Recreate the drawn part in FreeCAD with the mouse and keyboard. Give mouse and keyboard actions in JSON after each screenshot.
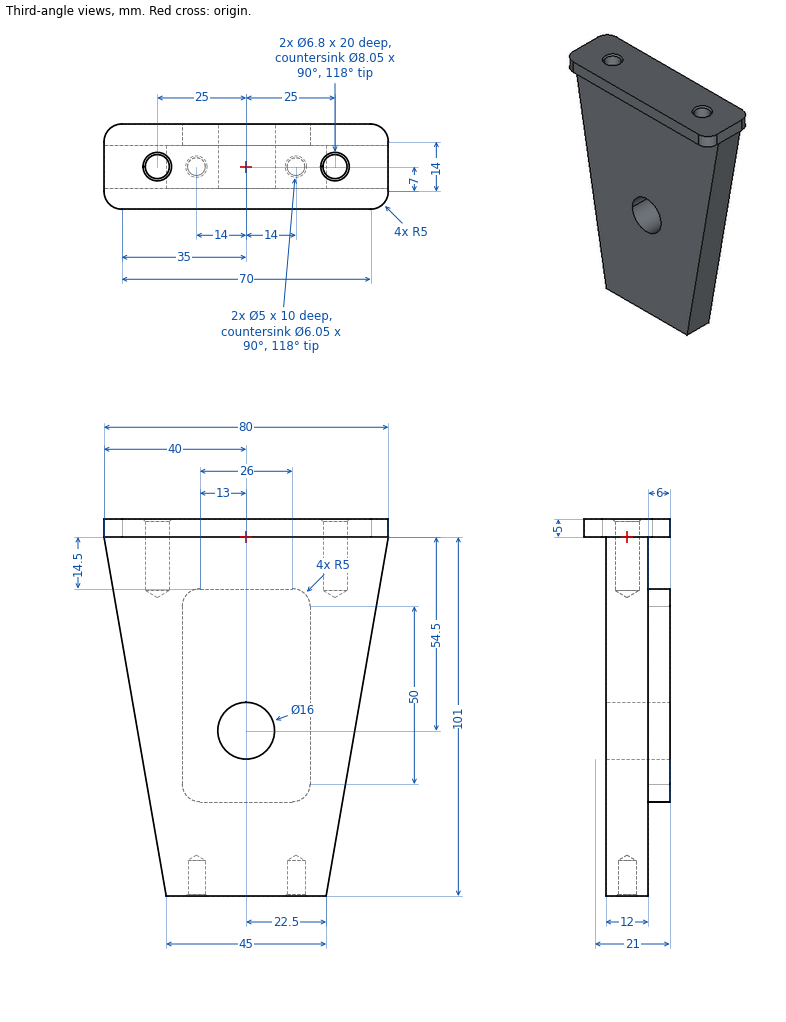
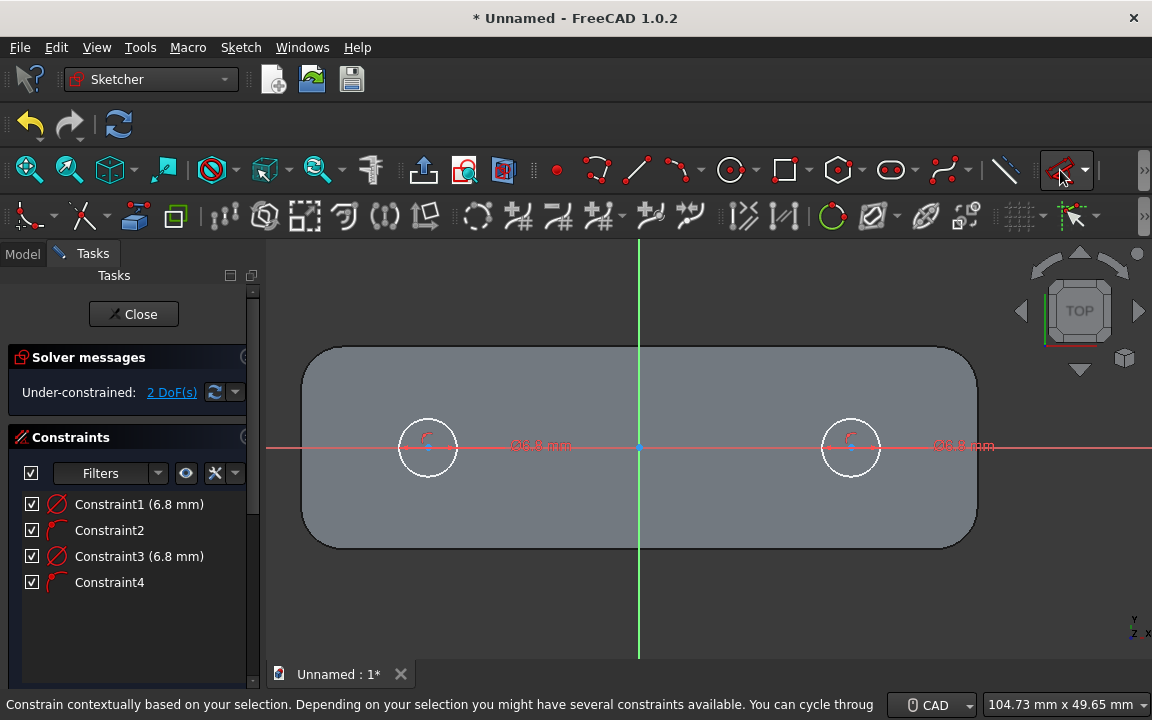
{"action": "left_click", "coordinate": [851, 448]}
{"action": "left_click", "coordinate": [745, 482]}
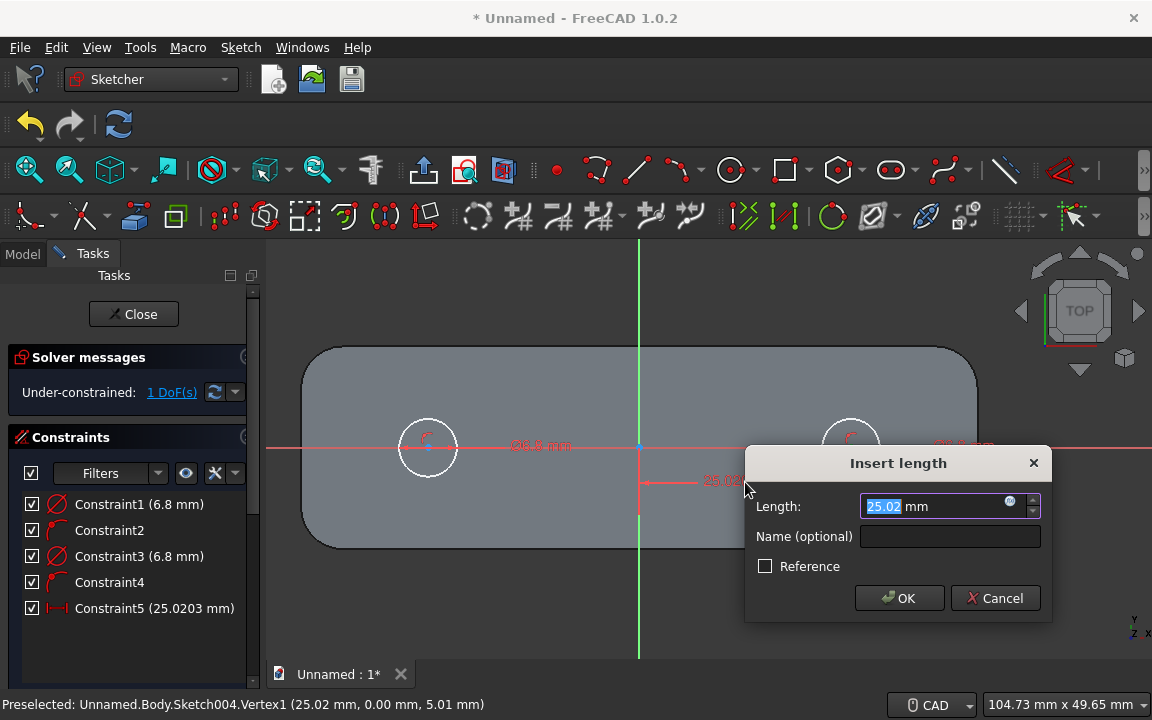
{"action": "type", "text": "25"}
{"action": "key", "text": "Return"}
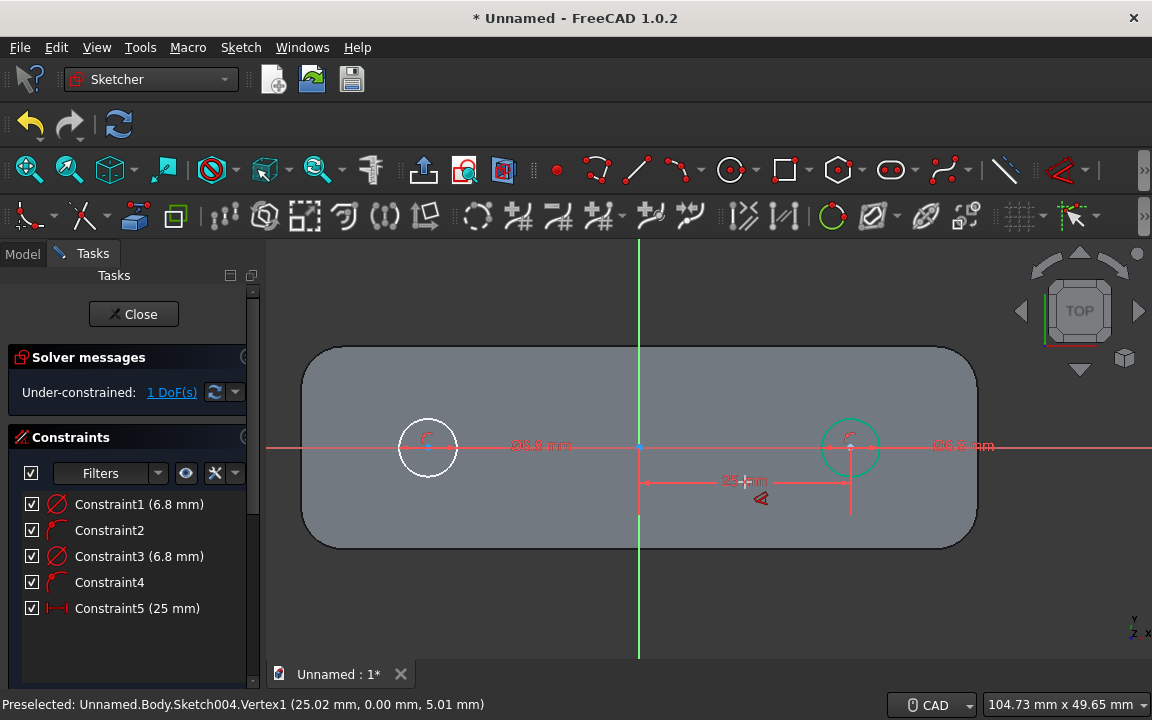
{"action": "left_click", "coordinate": [428, 448]}
{"action": "left_click", "coordinate": [534, 482]}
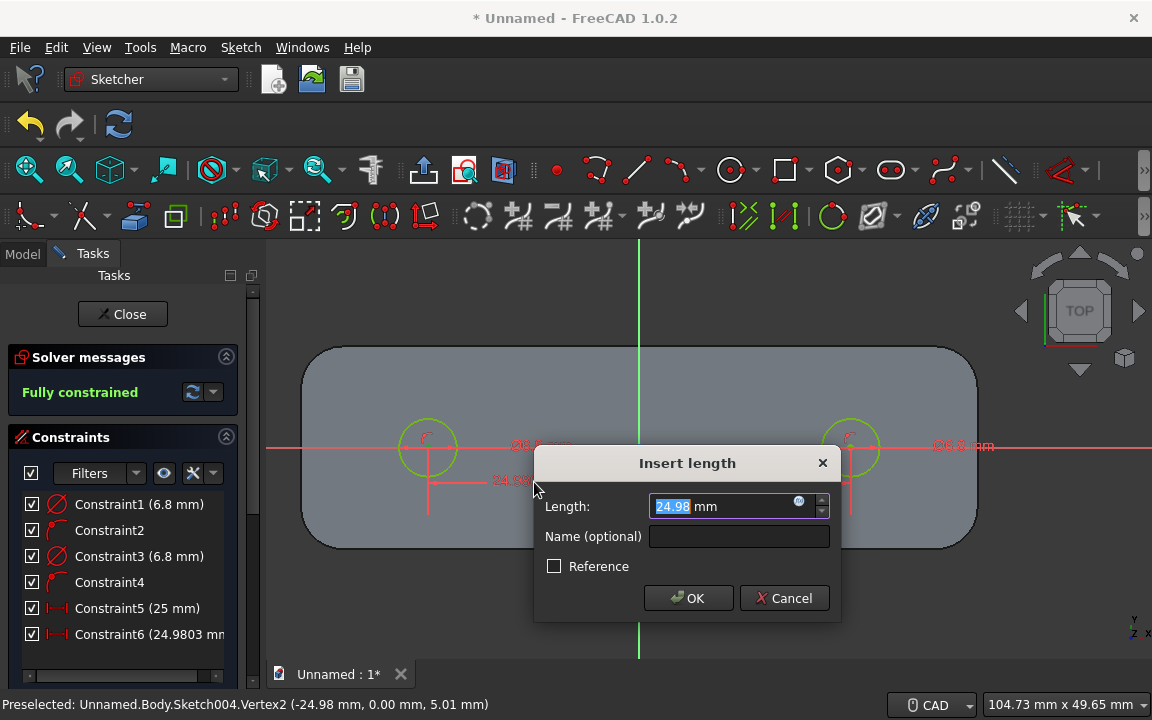
{"action": "type", "text": "25"}
{"action": "key", "text": "Return"}
{"action": "key", "text": "Escape"}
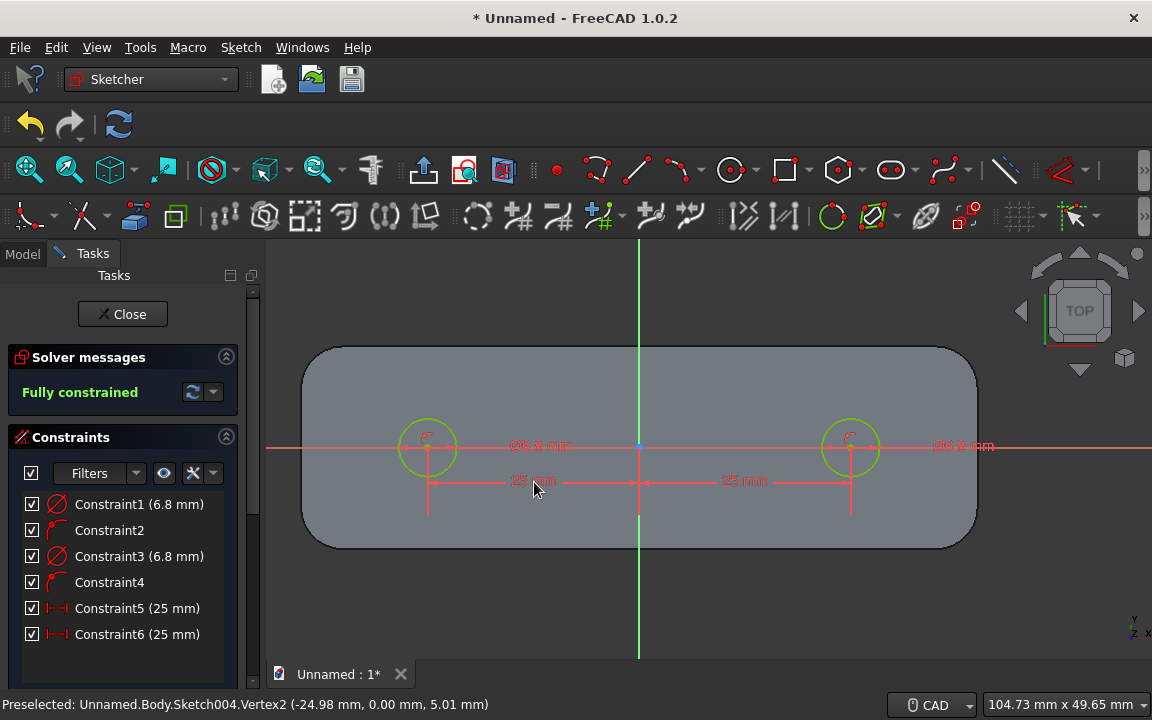
{"action": "left_click", "coordinate": [123, 314]}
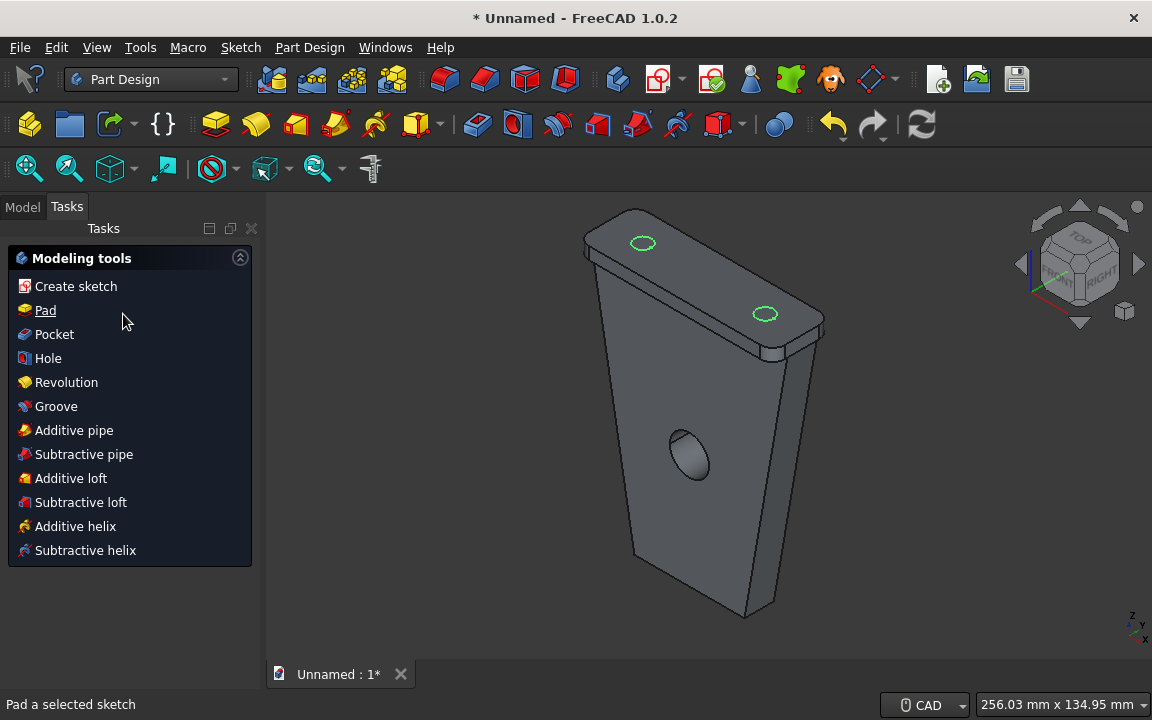
{"action": "left_click", "coordinate": [518, 124]}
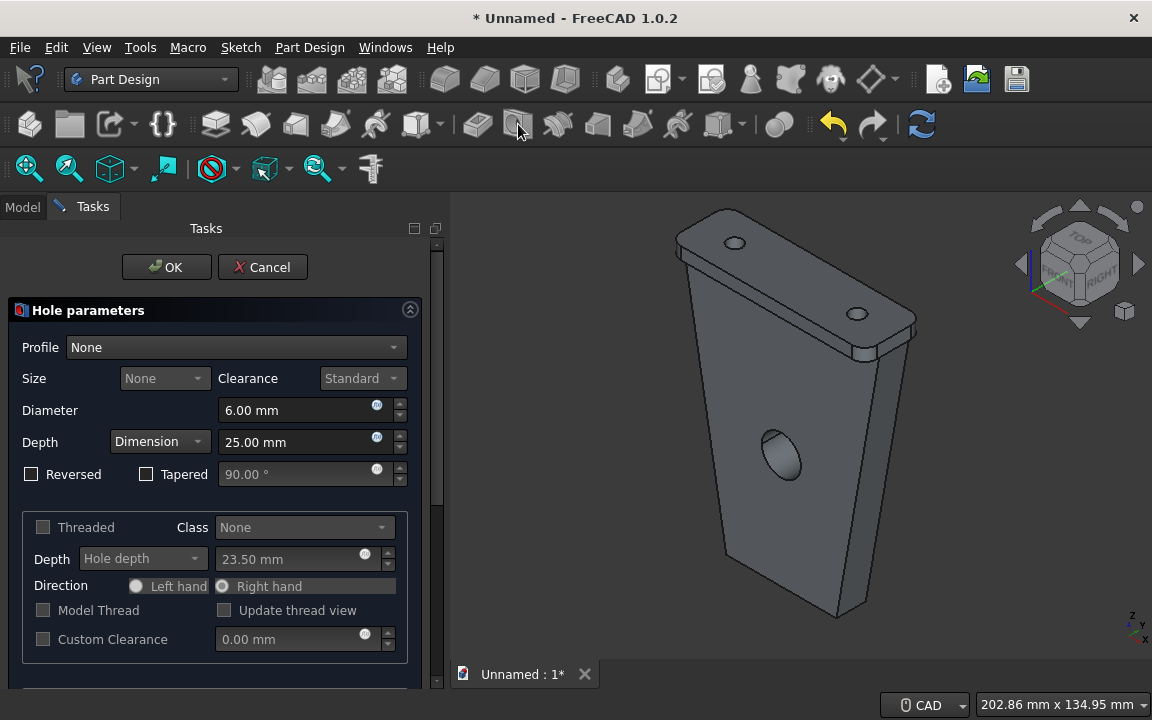
{"action": "triple_click", "coordinate": [305, 410]}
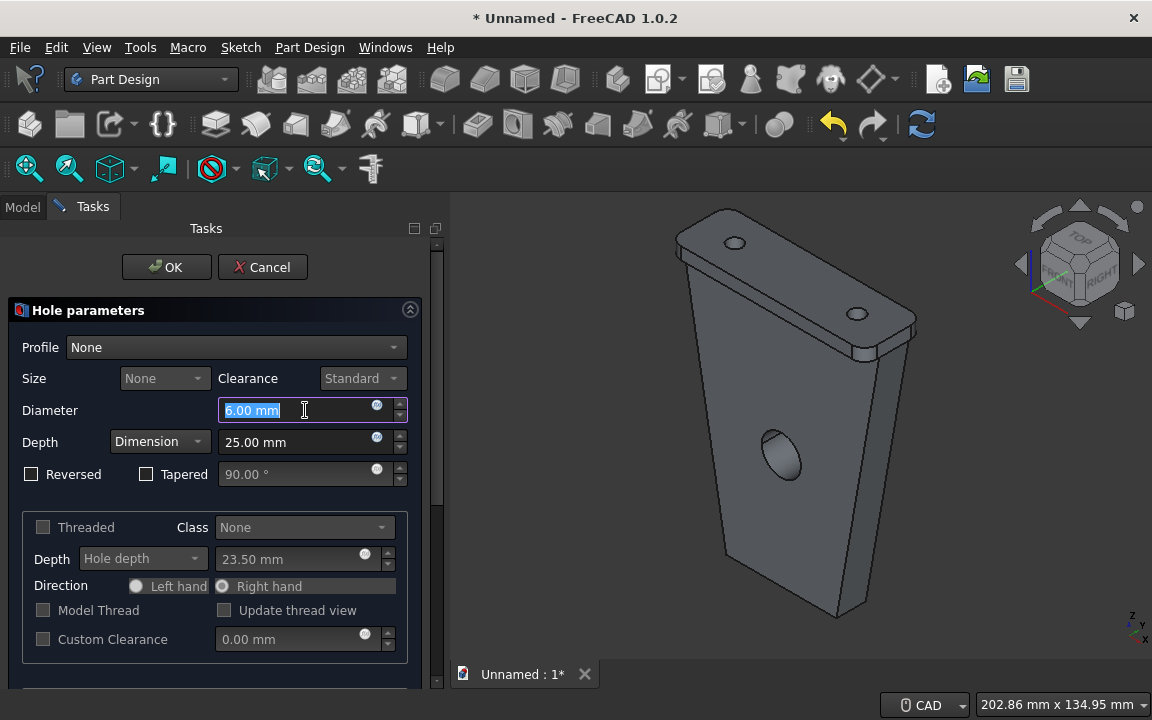
{"action": "type", "text": "6.8"}
{"action": "key", "text": "Tab"}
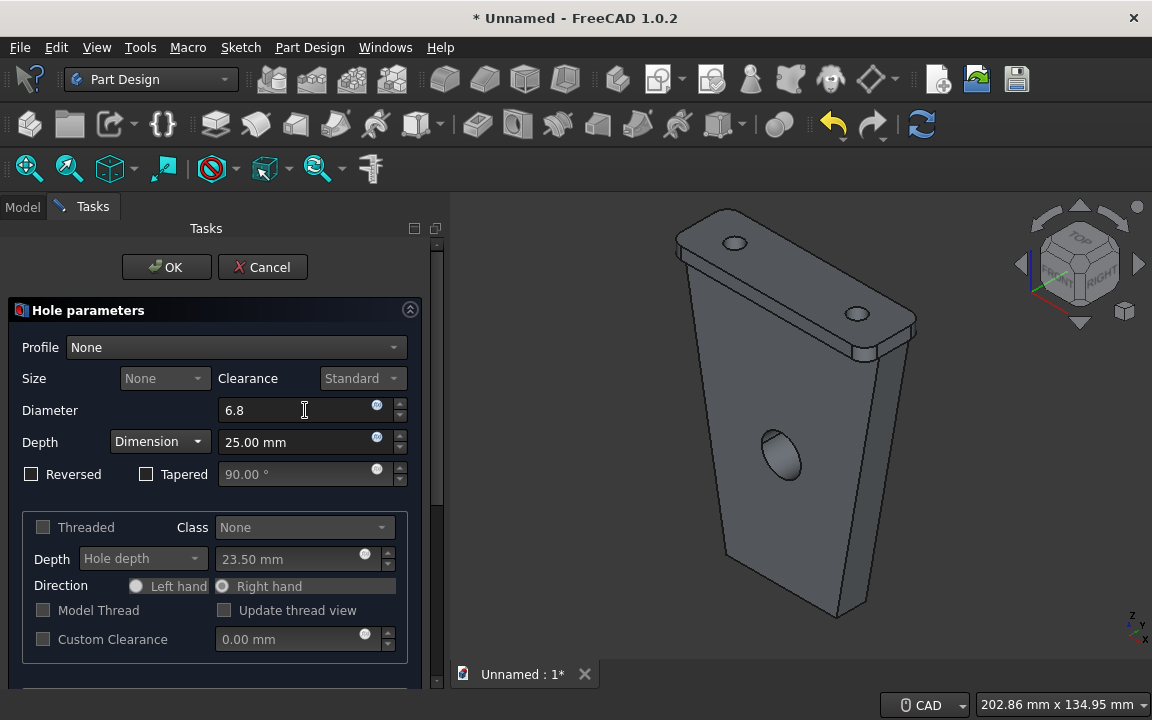
{"action": "triple_click", "coordinate": [305, 442]}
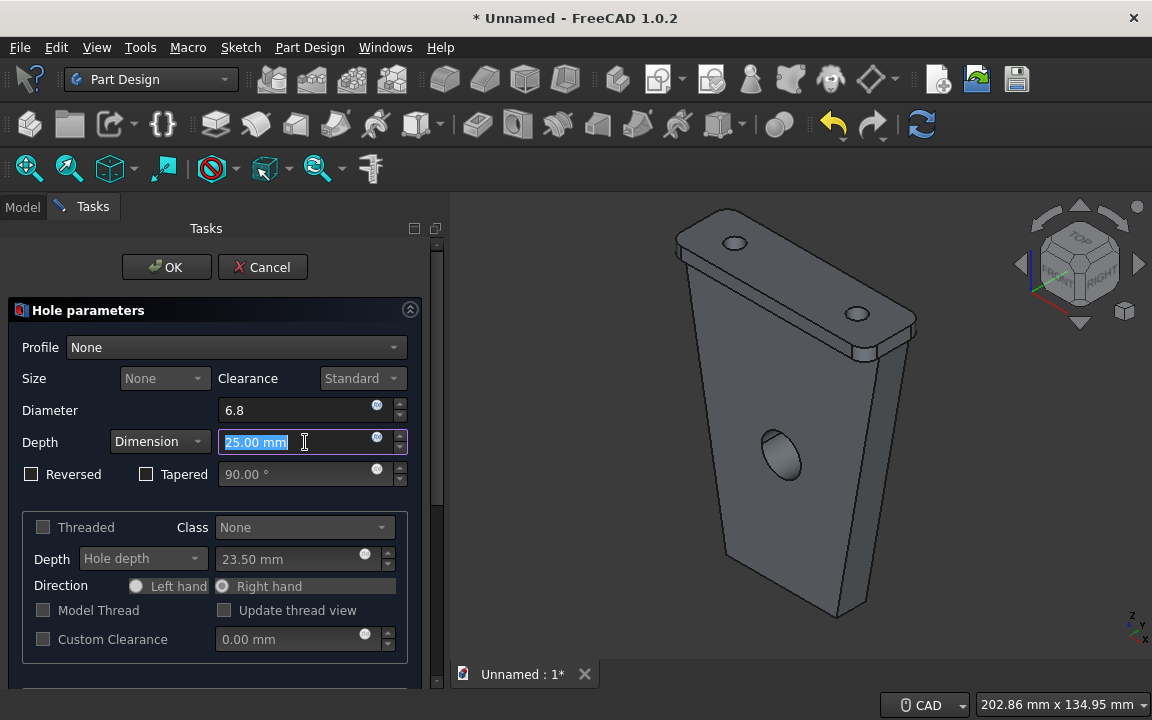
{"action": "type", "text": "20"}
{"action": "key", "text": "Tab"}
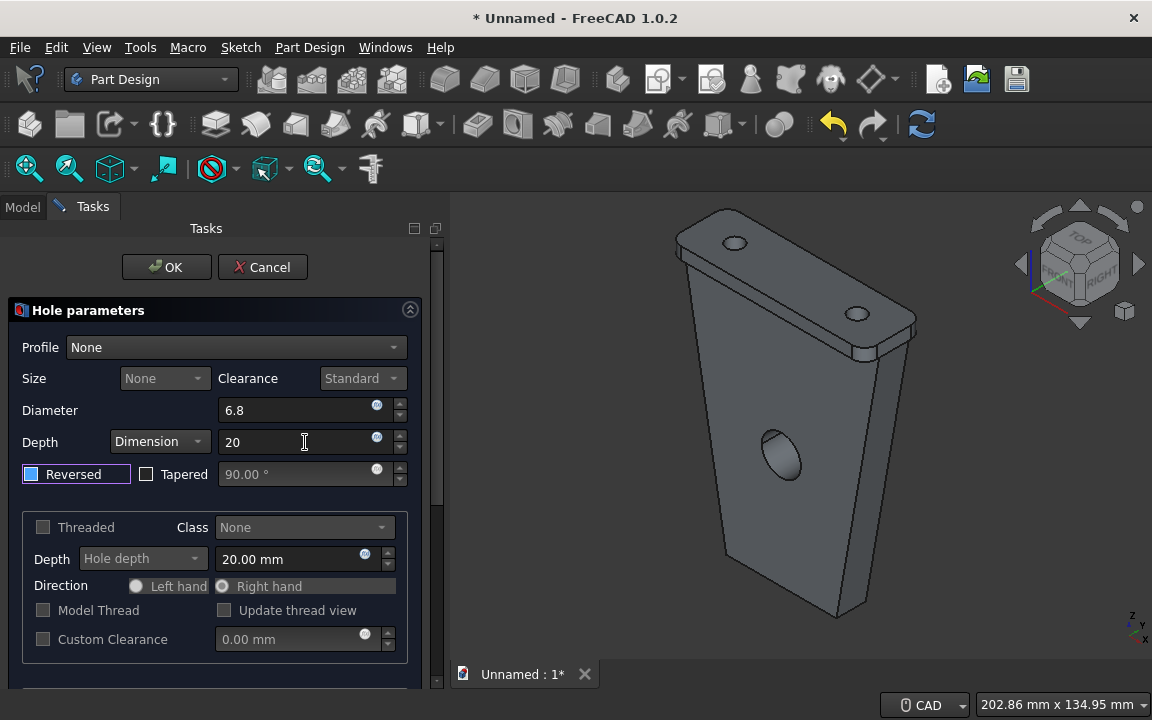
{"action": "scroll", "coordinate": [437, 463], "scroll_direction": "down", "scroll_amount": 2}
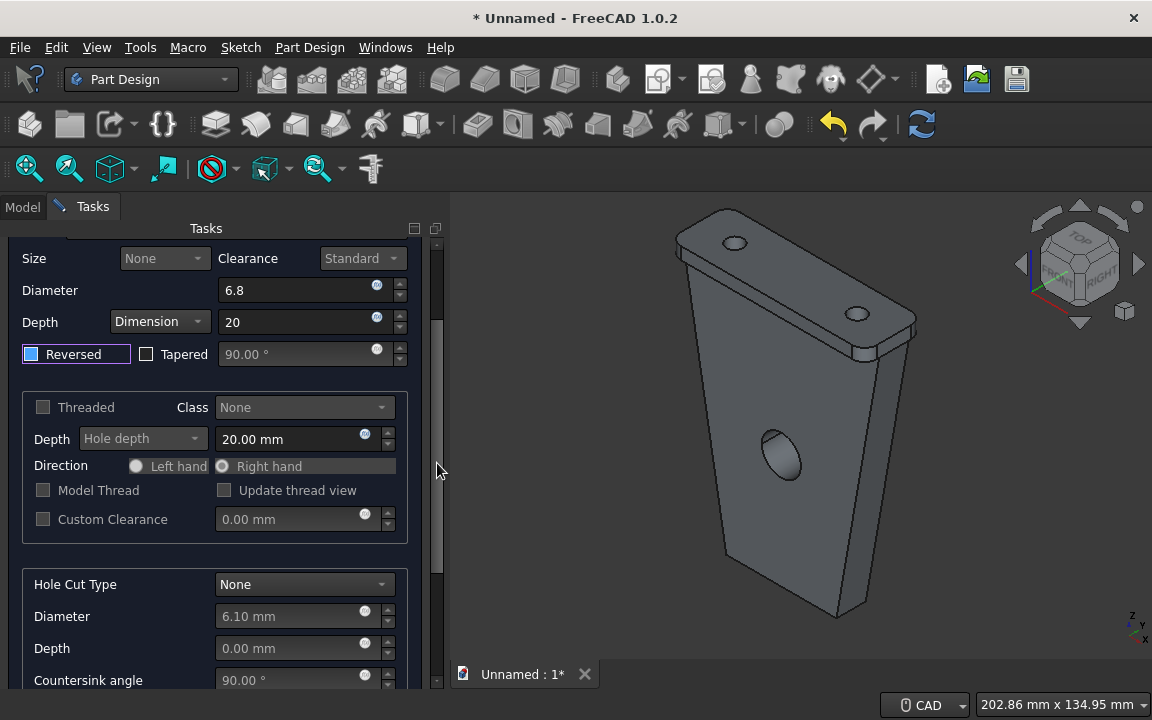
{"action": "left_click", "coordinate": [306, 584]}